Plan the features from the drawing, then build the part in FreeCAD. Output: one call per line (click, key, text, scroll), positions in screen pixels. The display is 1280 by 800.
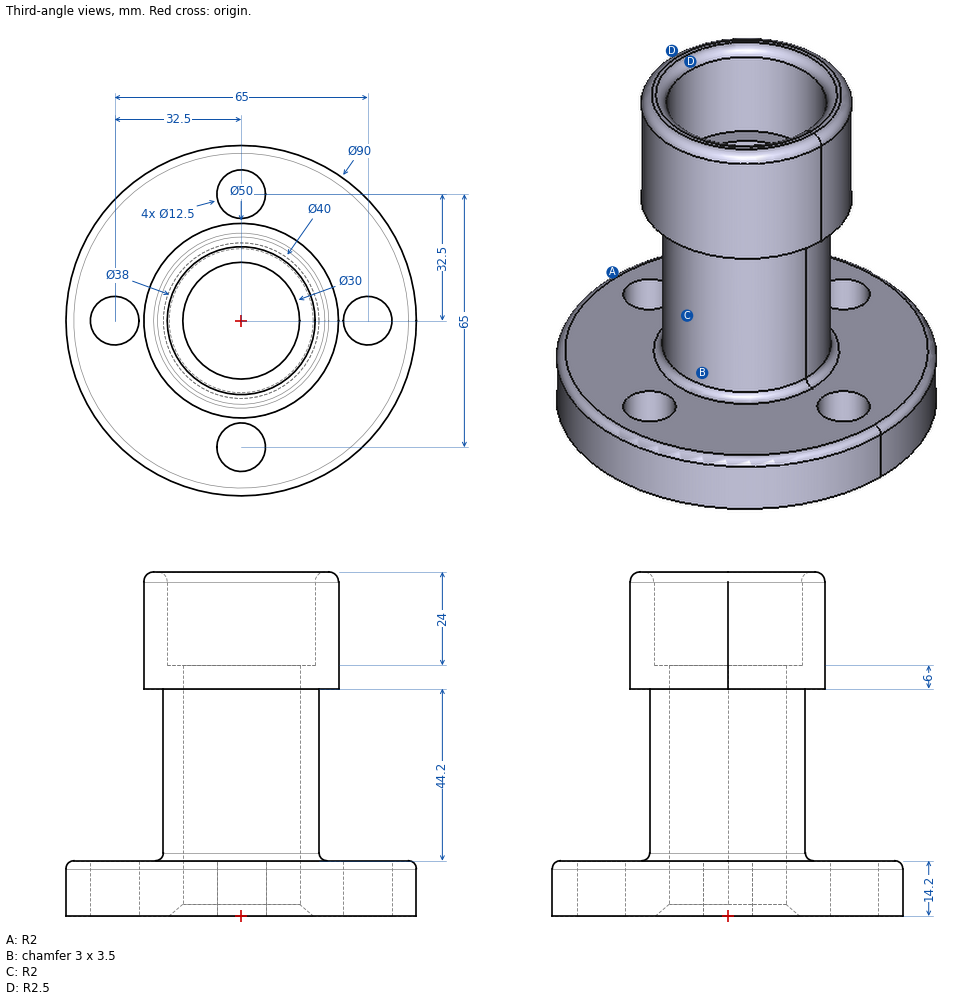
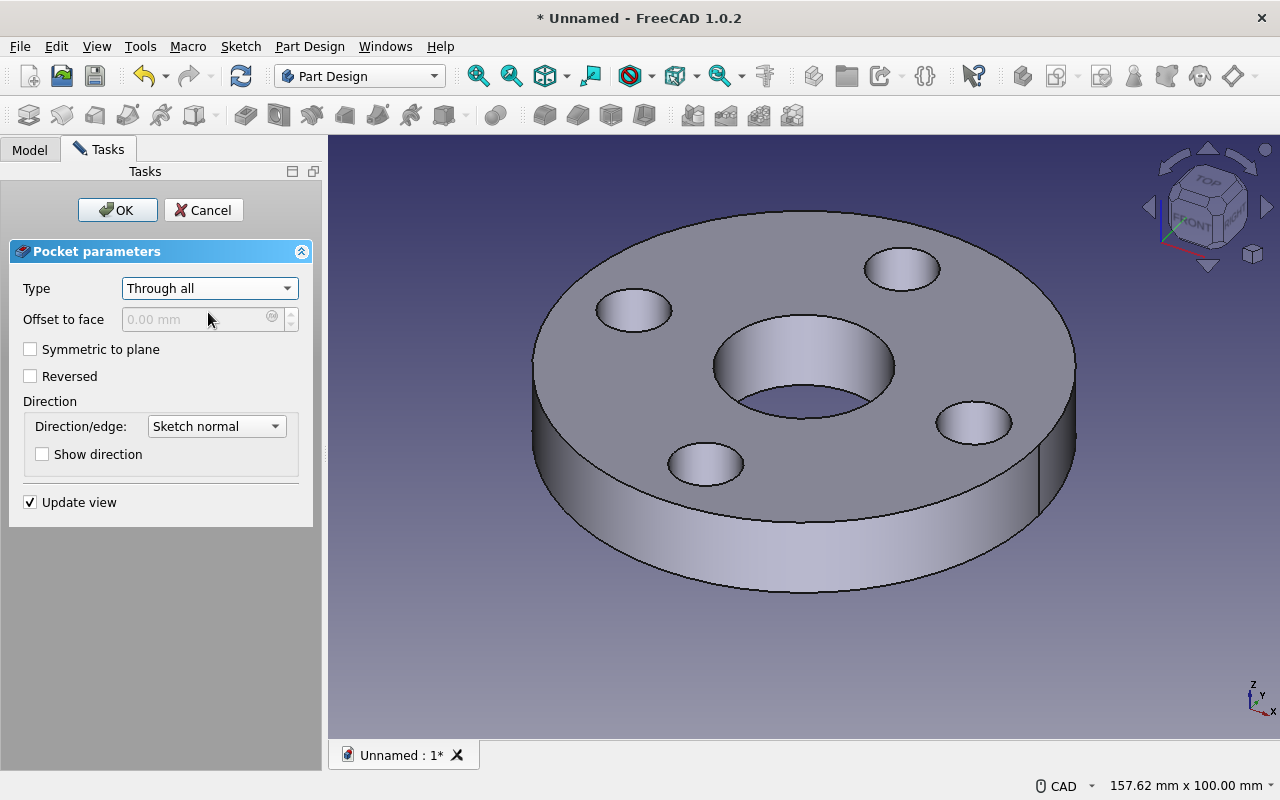
click(118, 210)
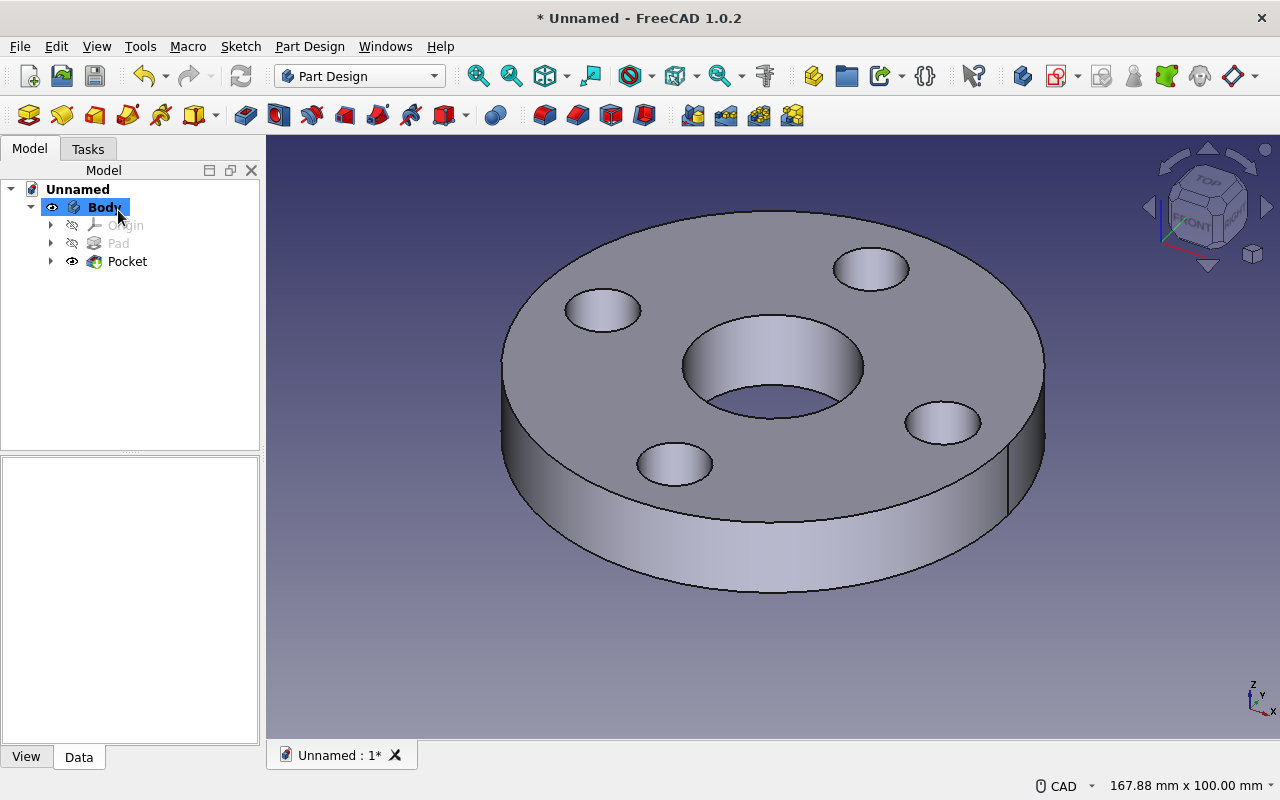
click(503, 382)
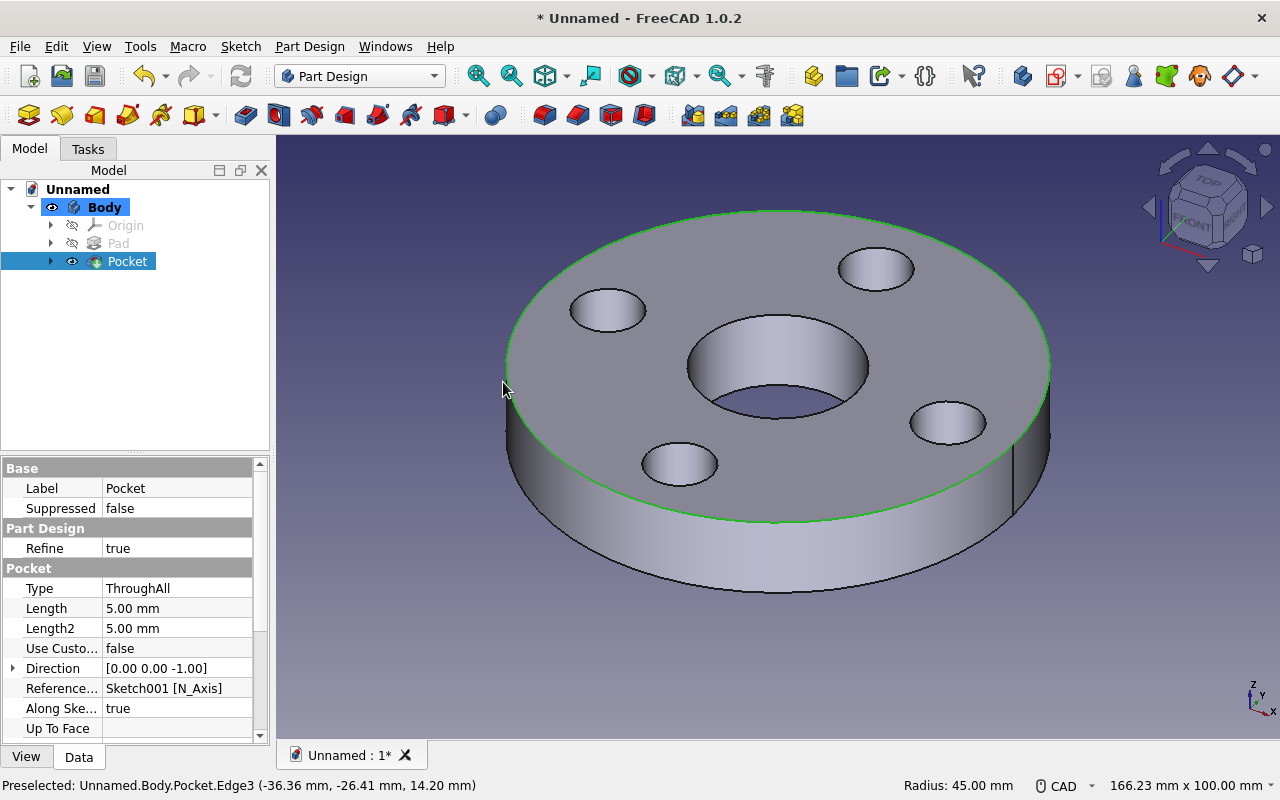
click(545, 116)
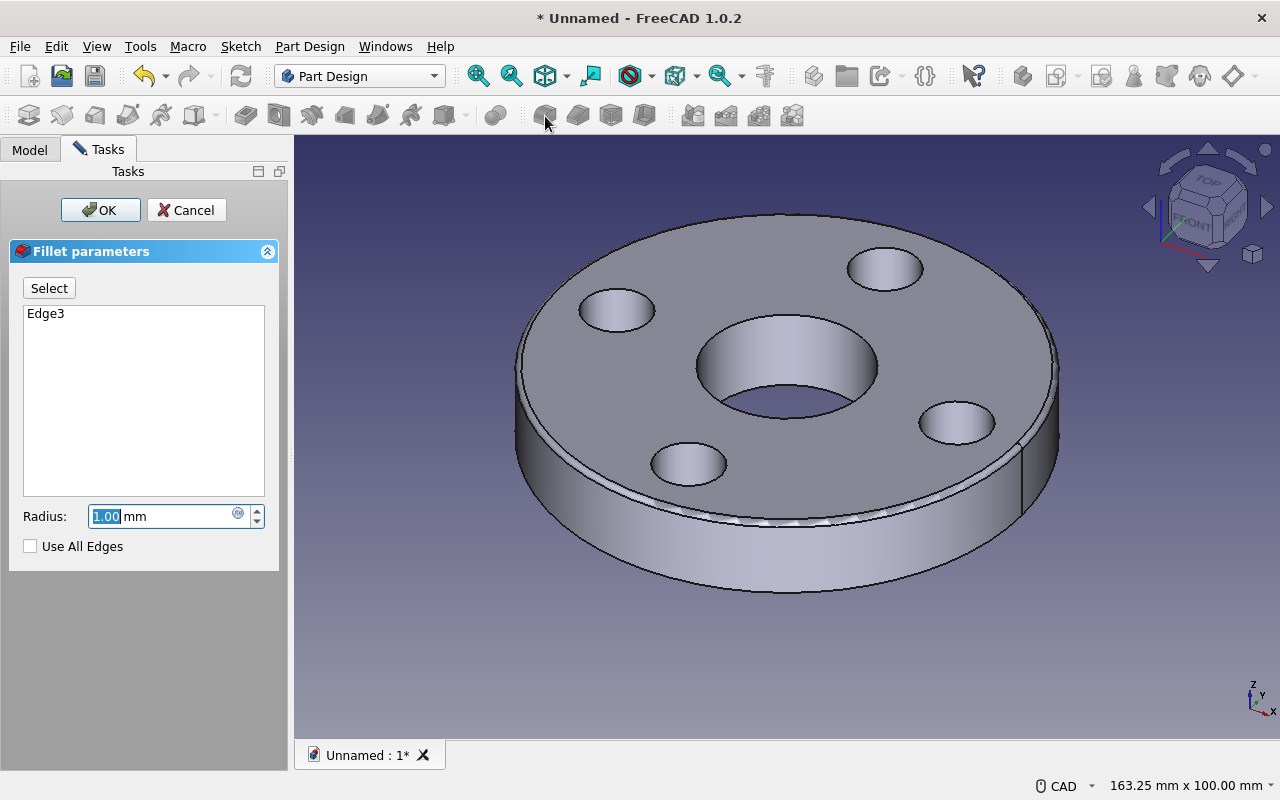
text(2)
key(Tab)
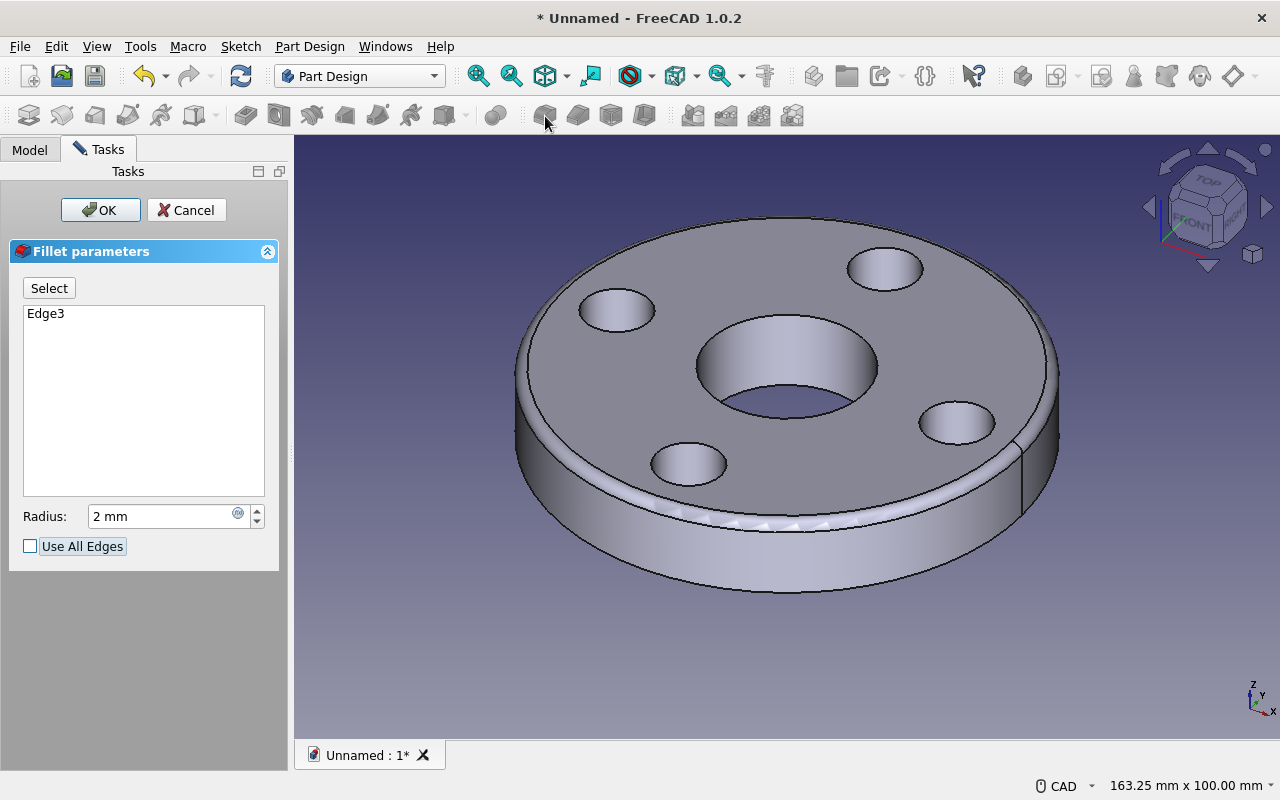
click(101, 210)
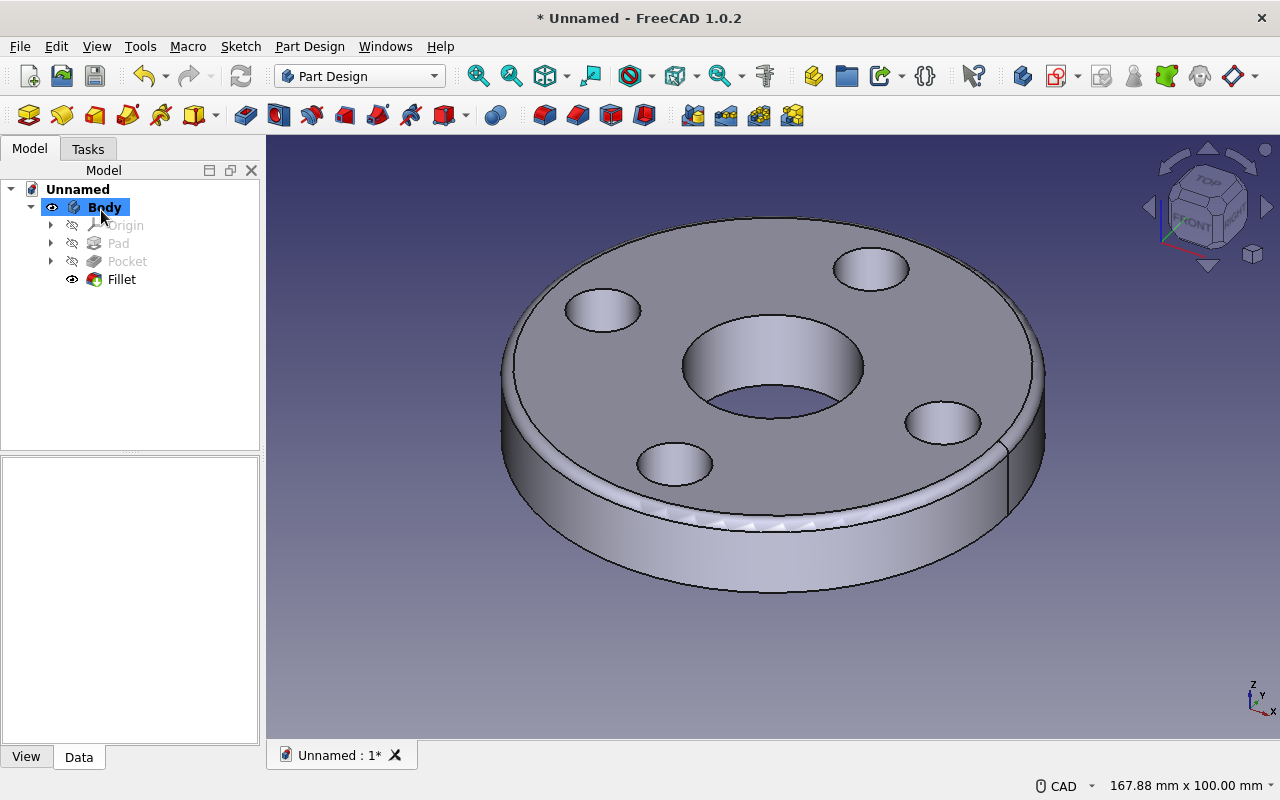
click(783, 271)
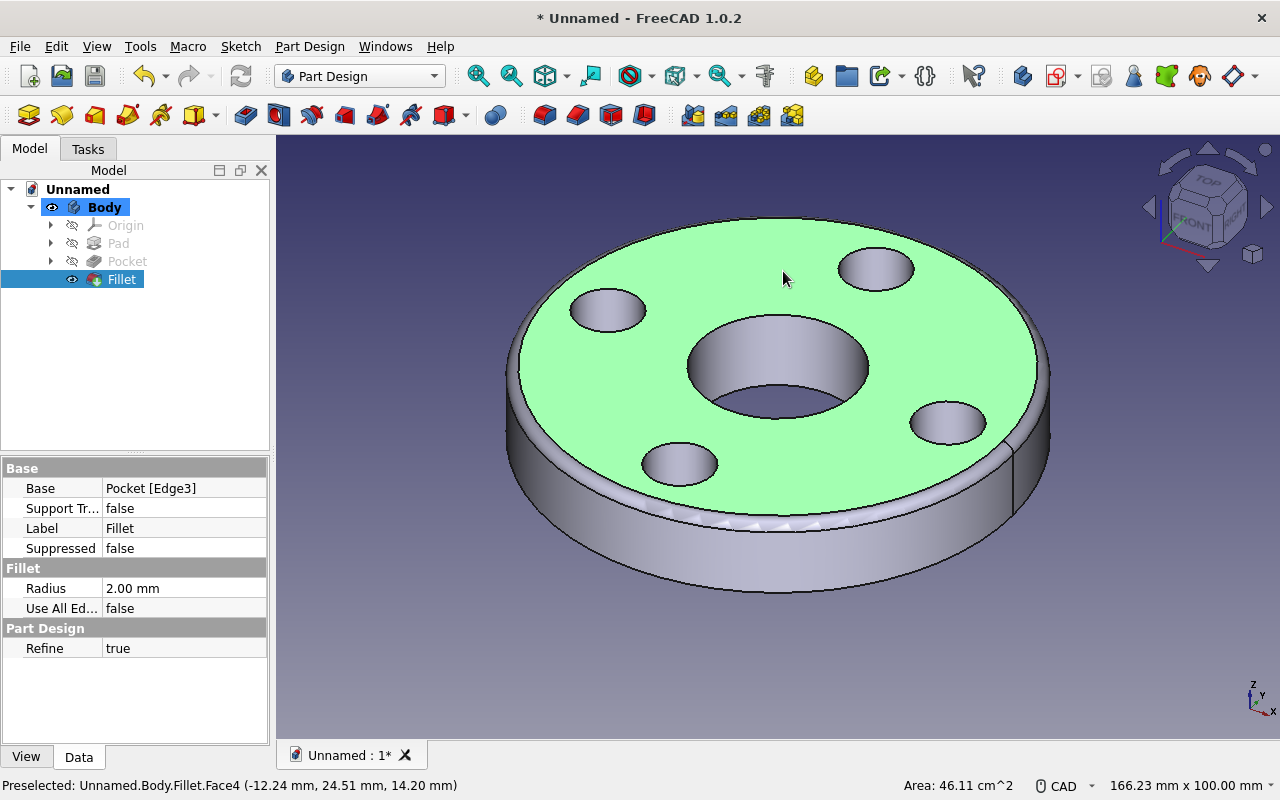
click(1056, 76)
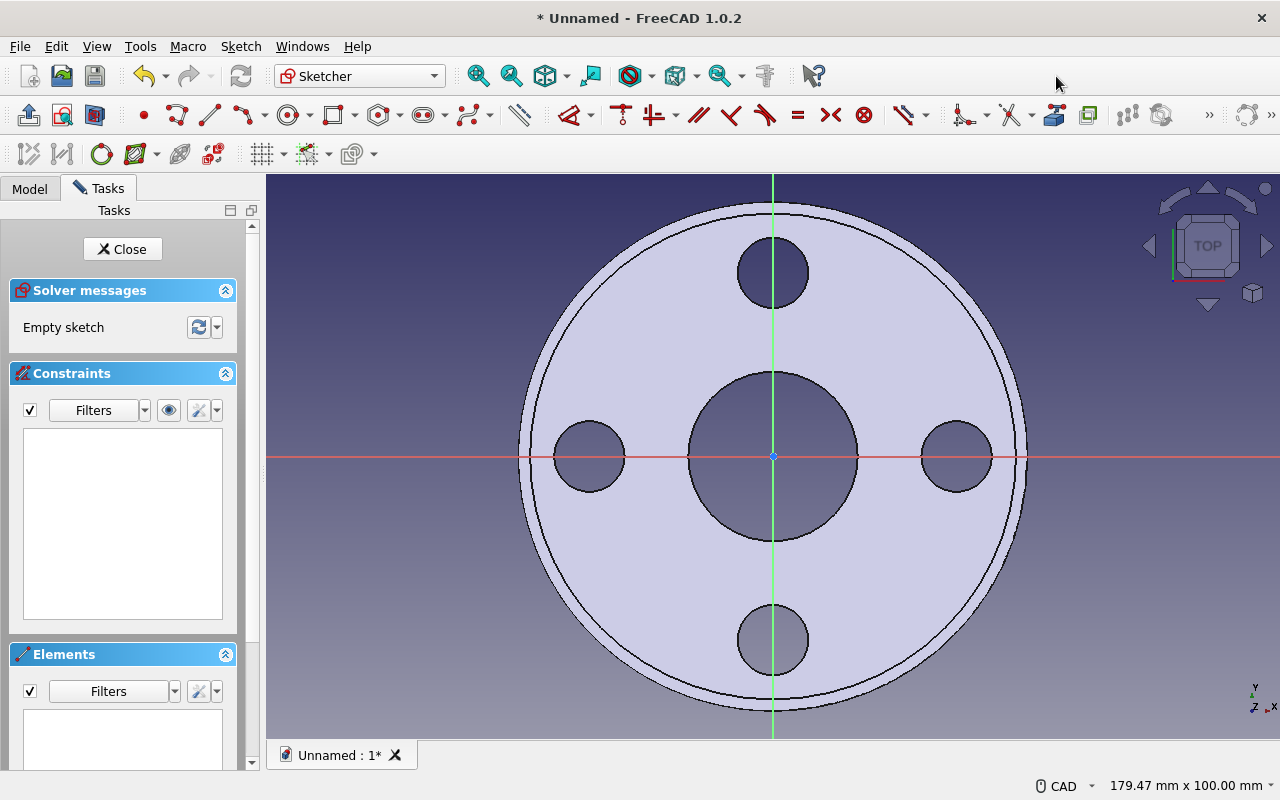
scroll(912, 456, up, 2)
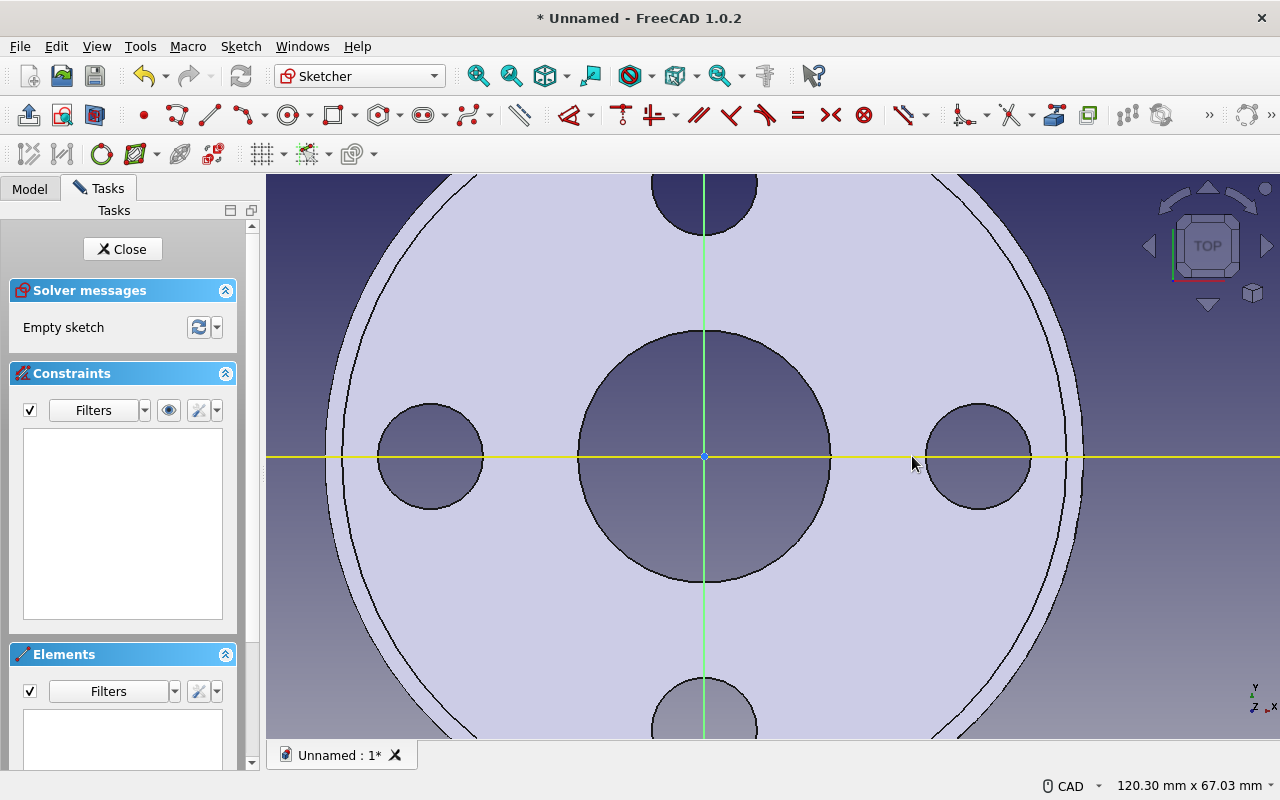
click(288, 116)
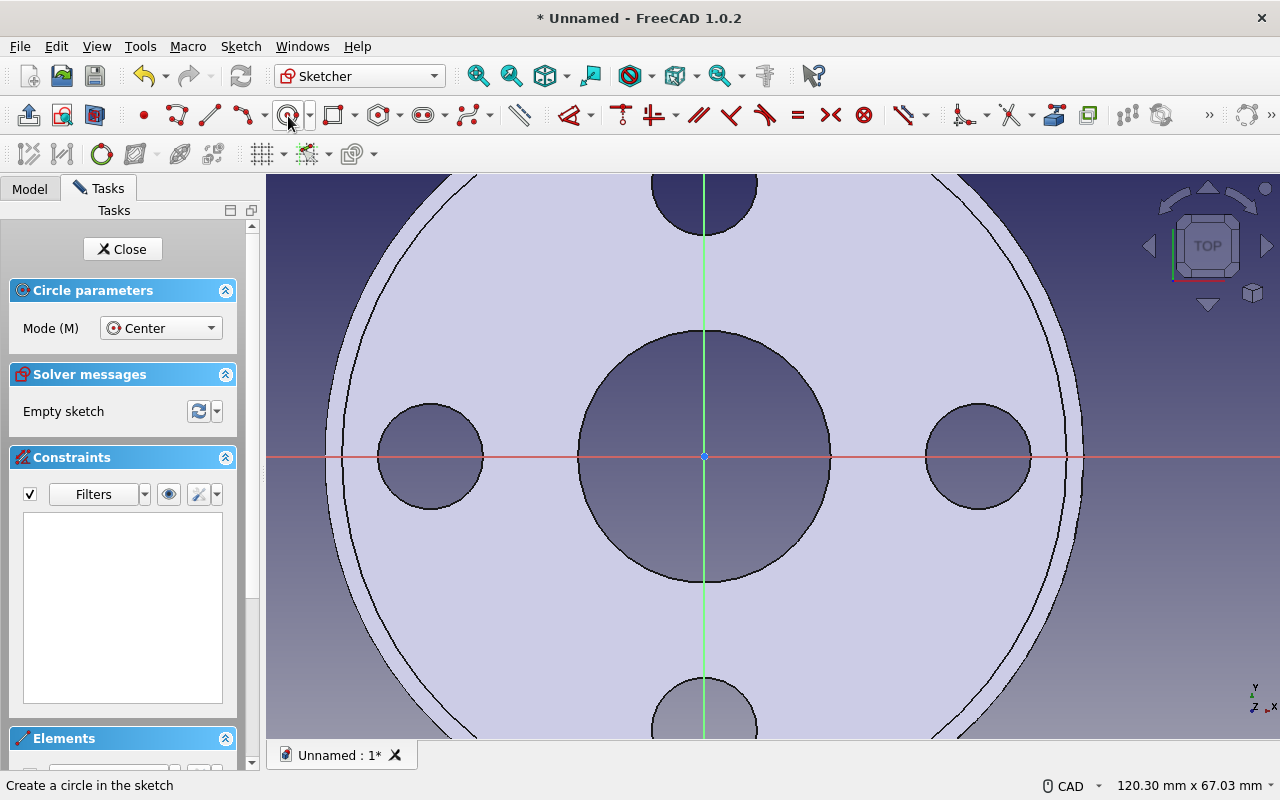
click(704, 456)
move(824, 337)